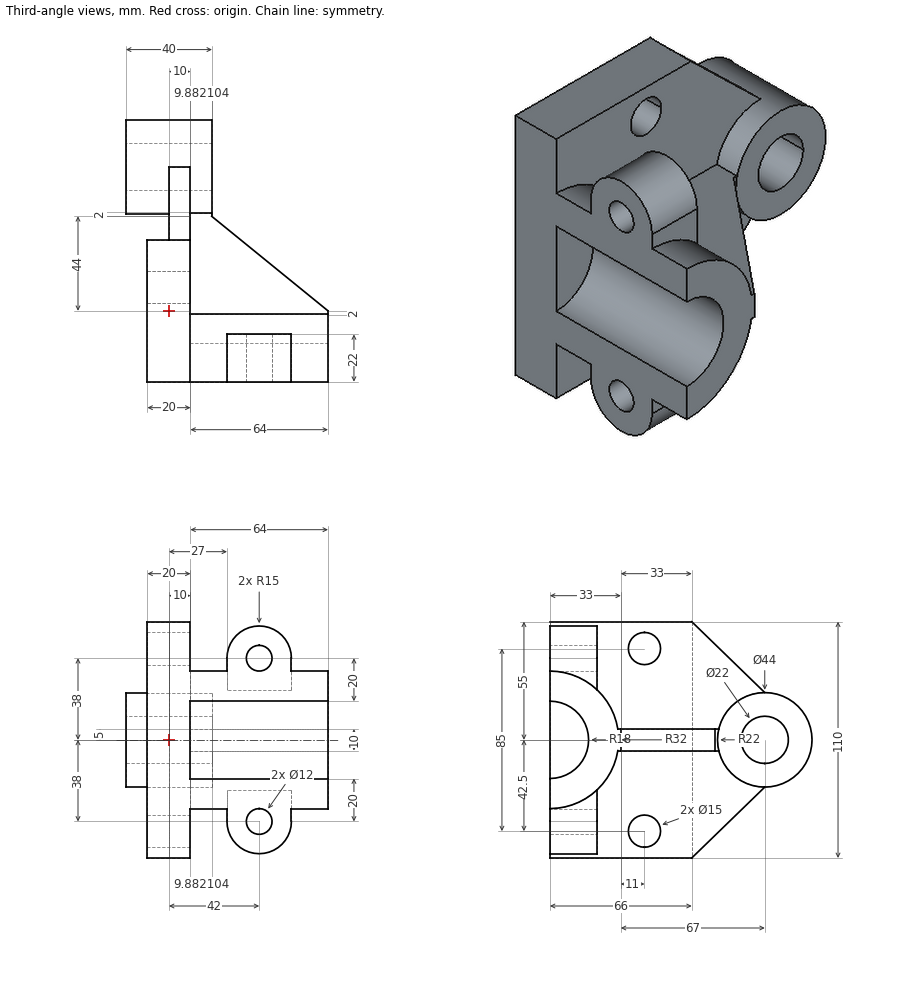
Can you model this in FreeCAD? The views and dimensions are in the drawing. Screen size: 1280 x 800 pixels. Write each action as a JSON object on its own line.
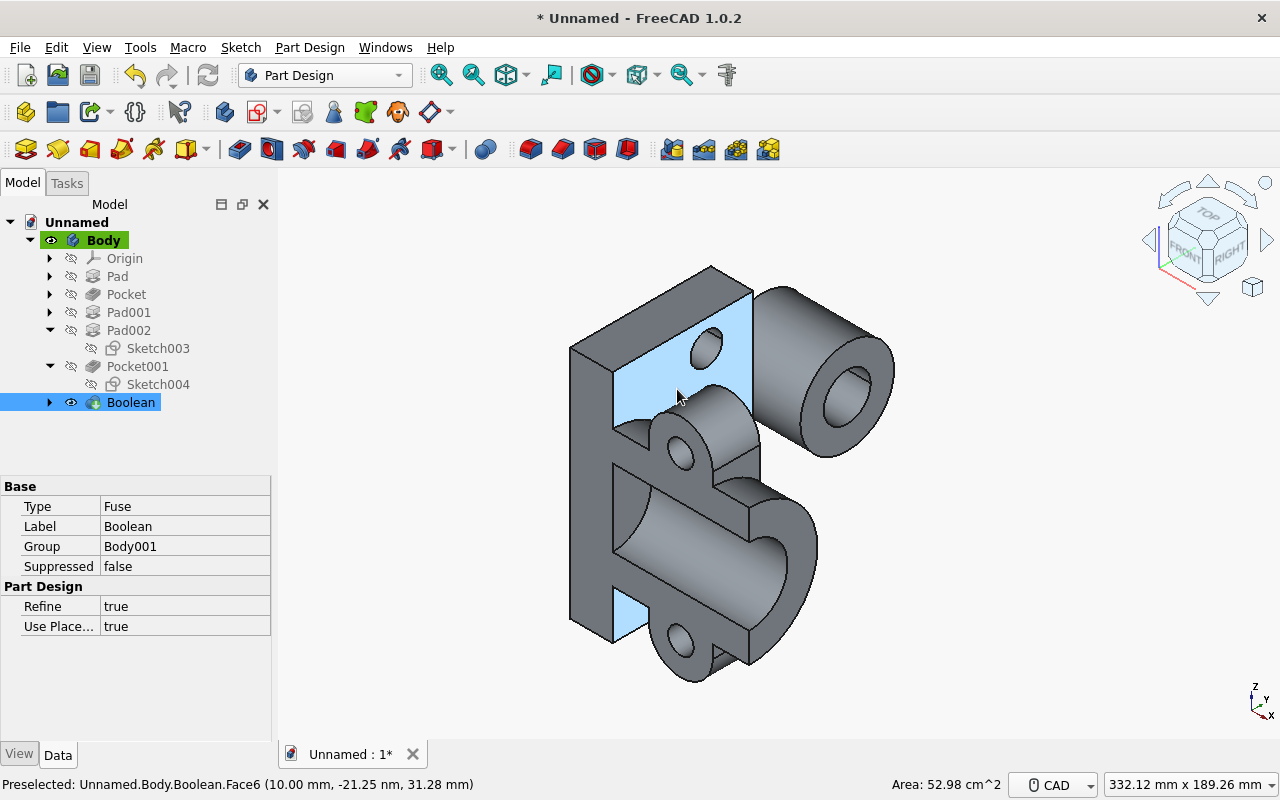
{"action": "left_click", "coordinate": [258, 112]}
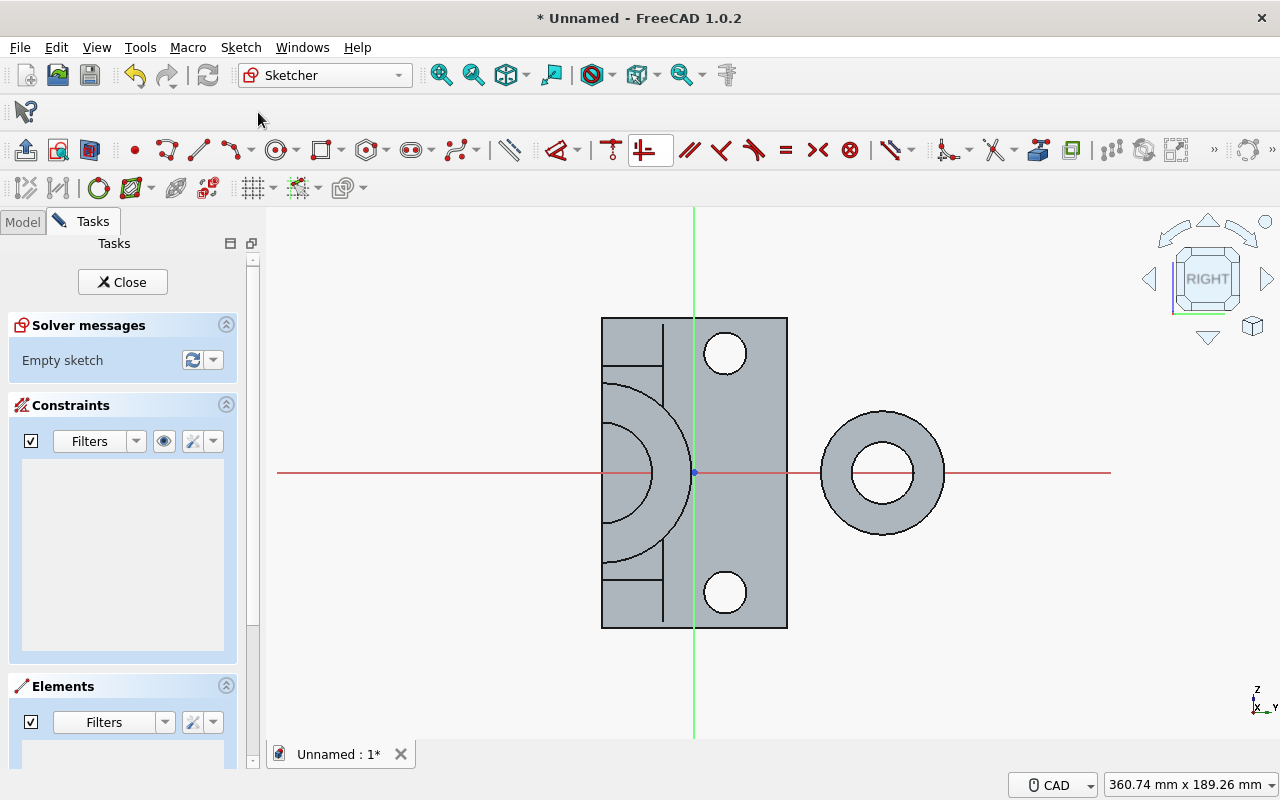
{"action": "left_click", "coordinate": [168, 150]}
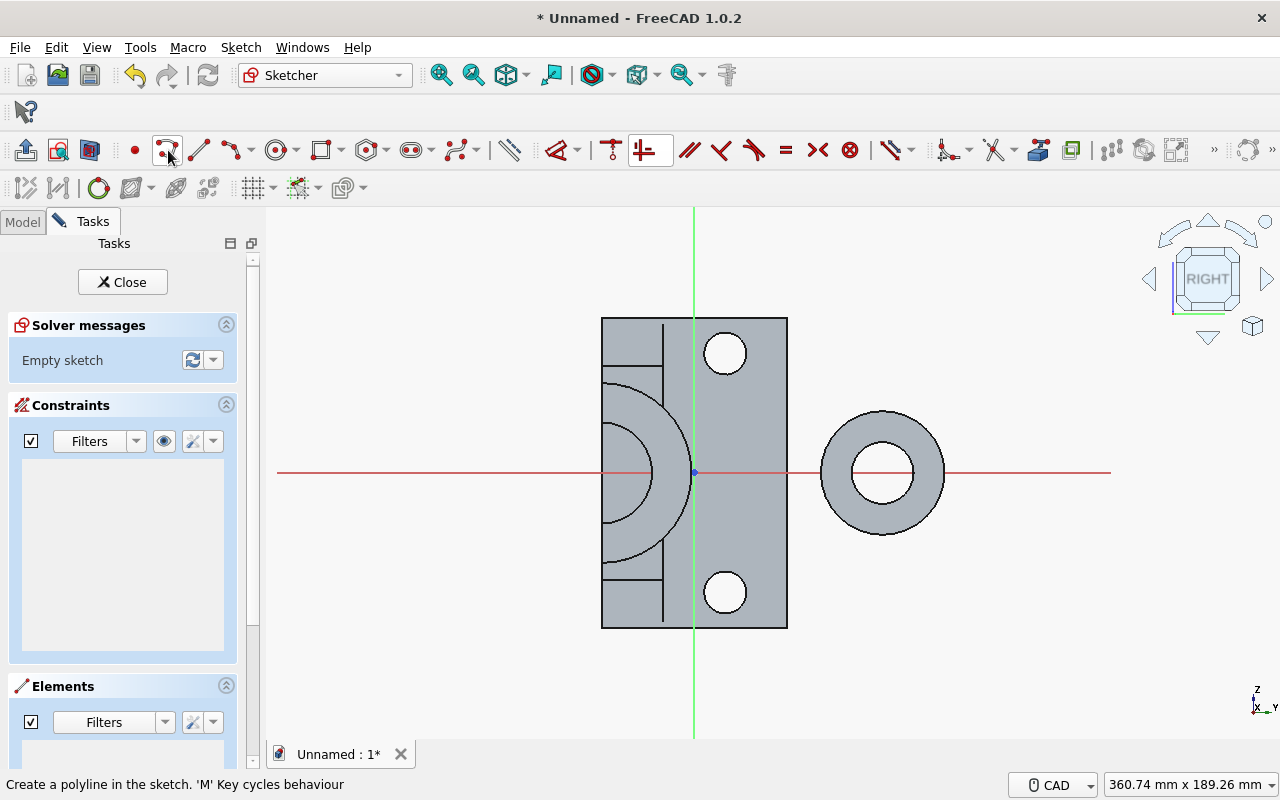
{"action": "left_click", "coordinate": [883, 411]}
{"action": "left_click", "coordinate": [787, 318]}
{"action": "left_click", "coordinate": [787, 628]}
{"action": "left_click", "coordinate": [883, 535]}
{"action": "right_click", "coordinate": [883, 535]}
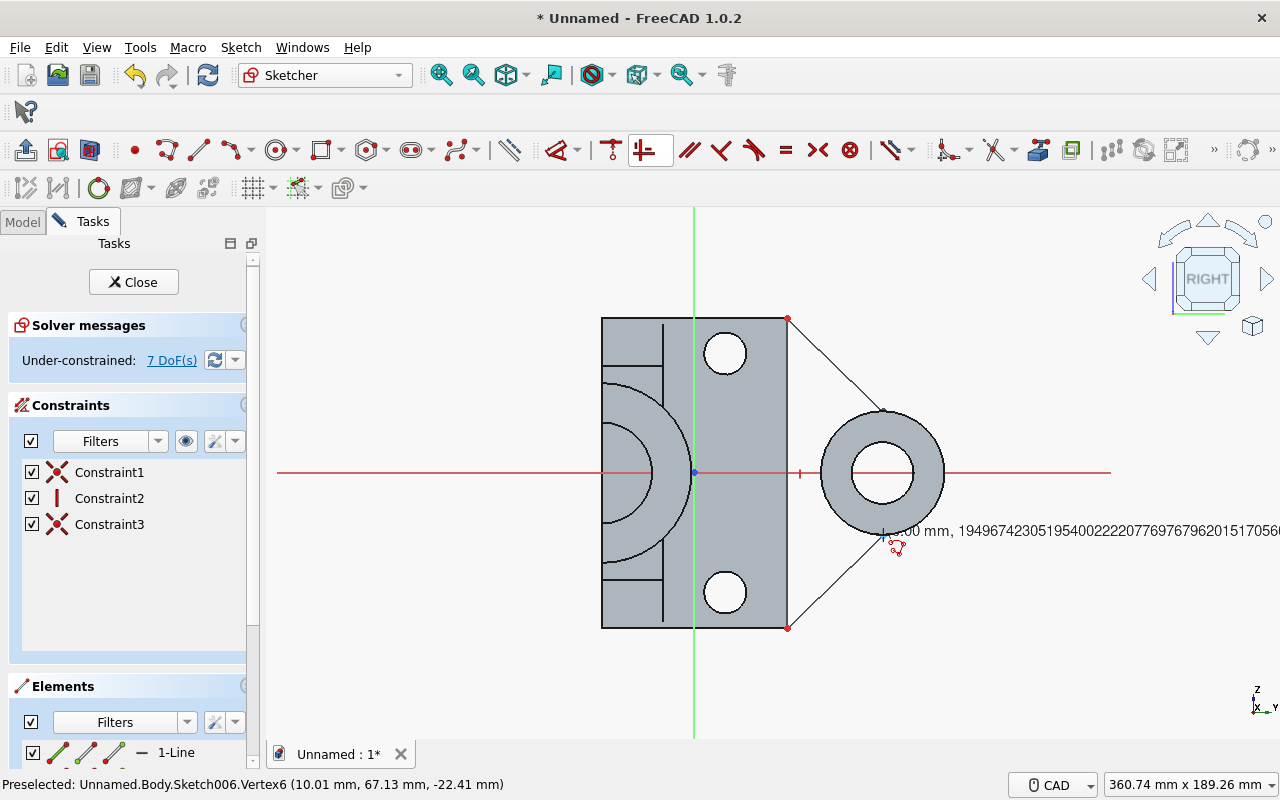
{"action": "left_click", "coordinate": [232, 150]}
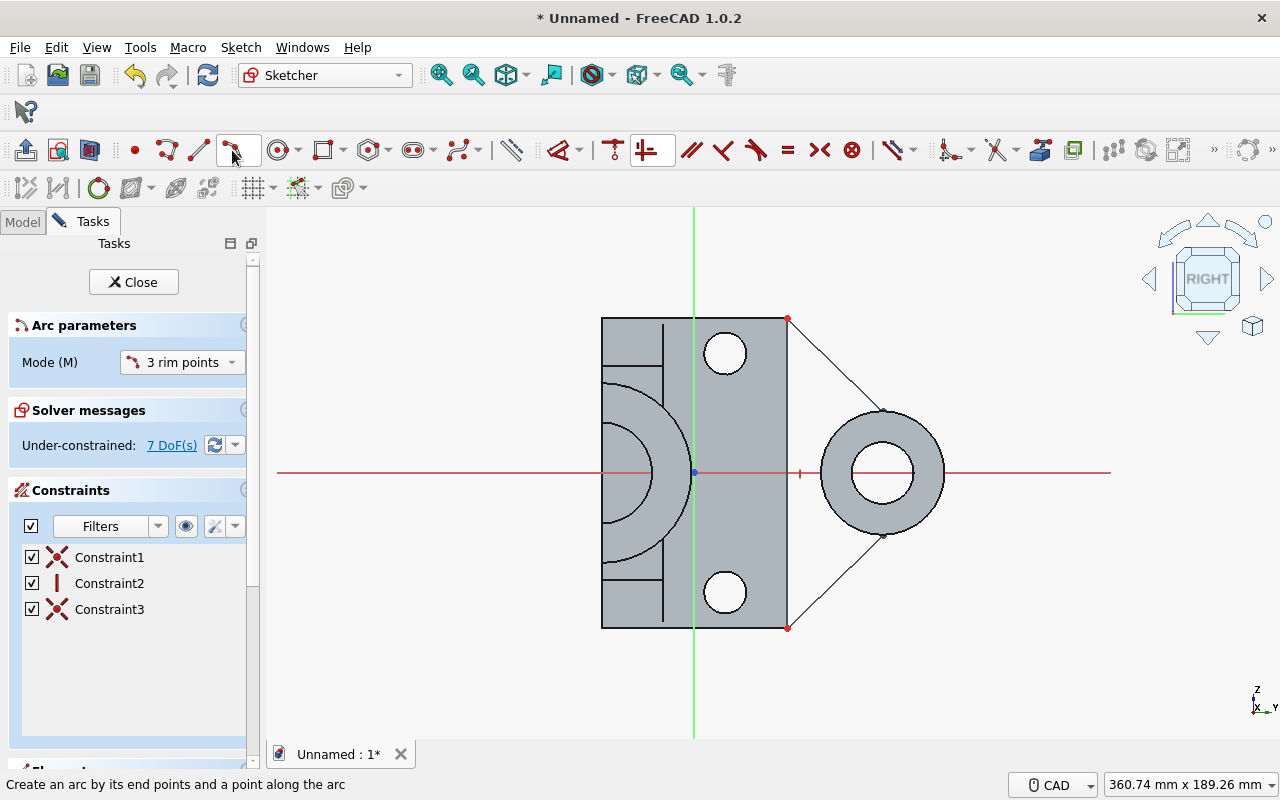
{"action": "left_click", "coordinate": [883, 536]}
{"action": "left_click", "coordinate": [883, 412]}
{"action": "left_click", "coordinate": [824, 454]}
{"action": "key", "text": "Escape"}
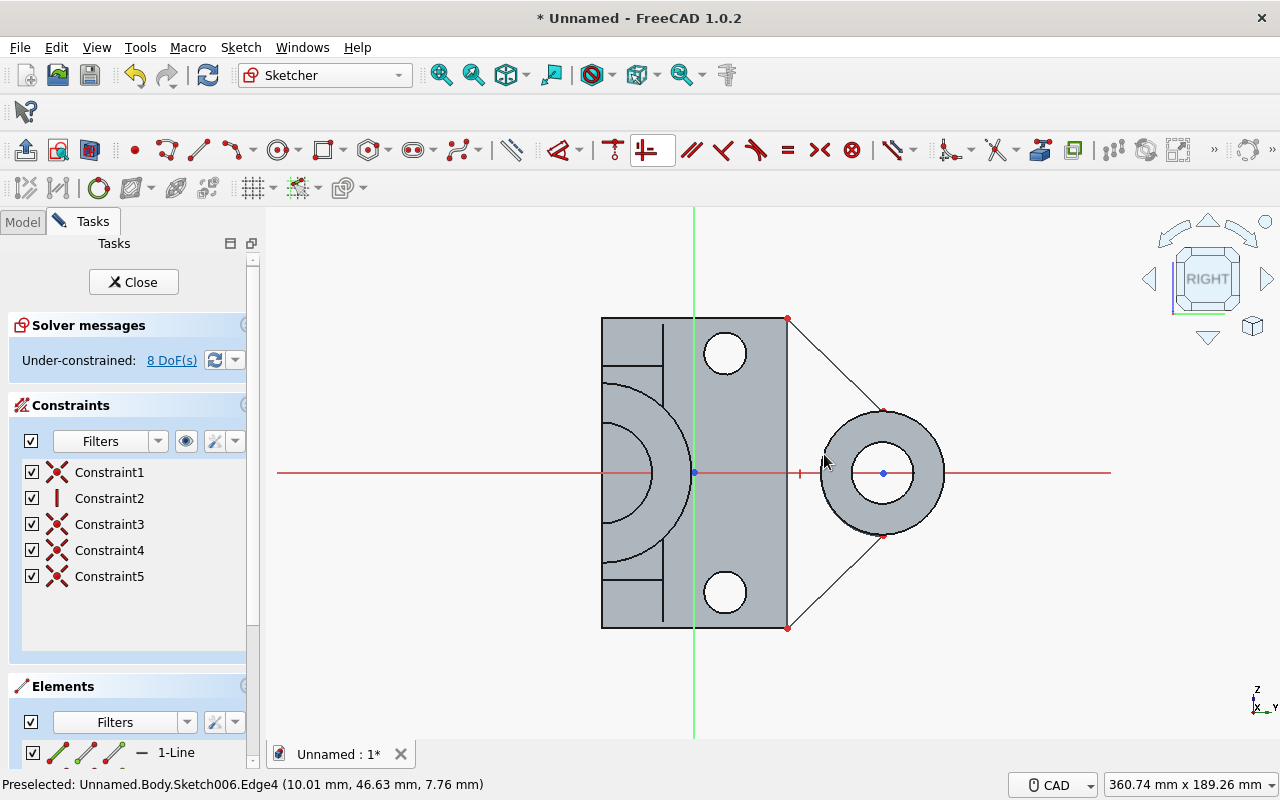
{"action": "left_click", "coordinate": [883, 474]}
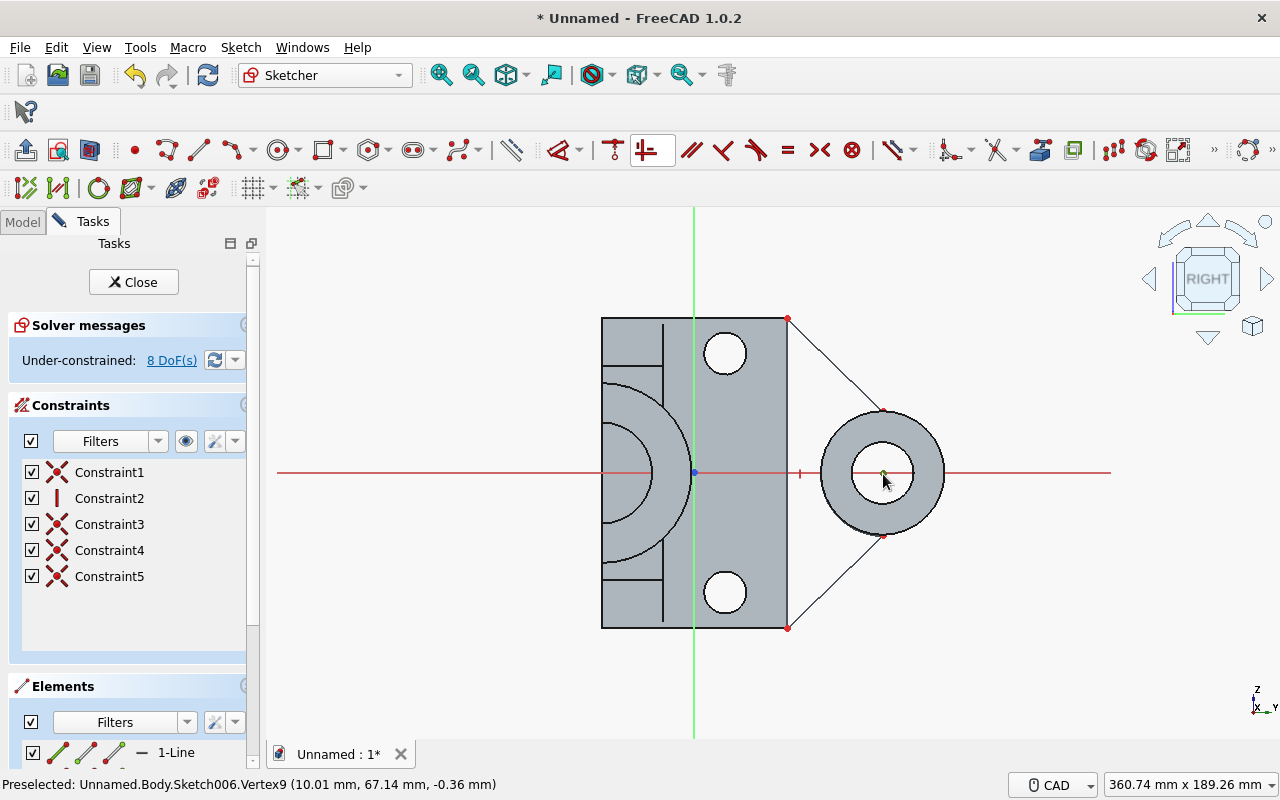
{"action": "left_click", "coordinate": [353, 473]}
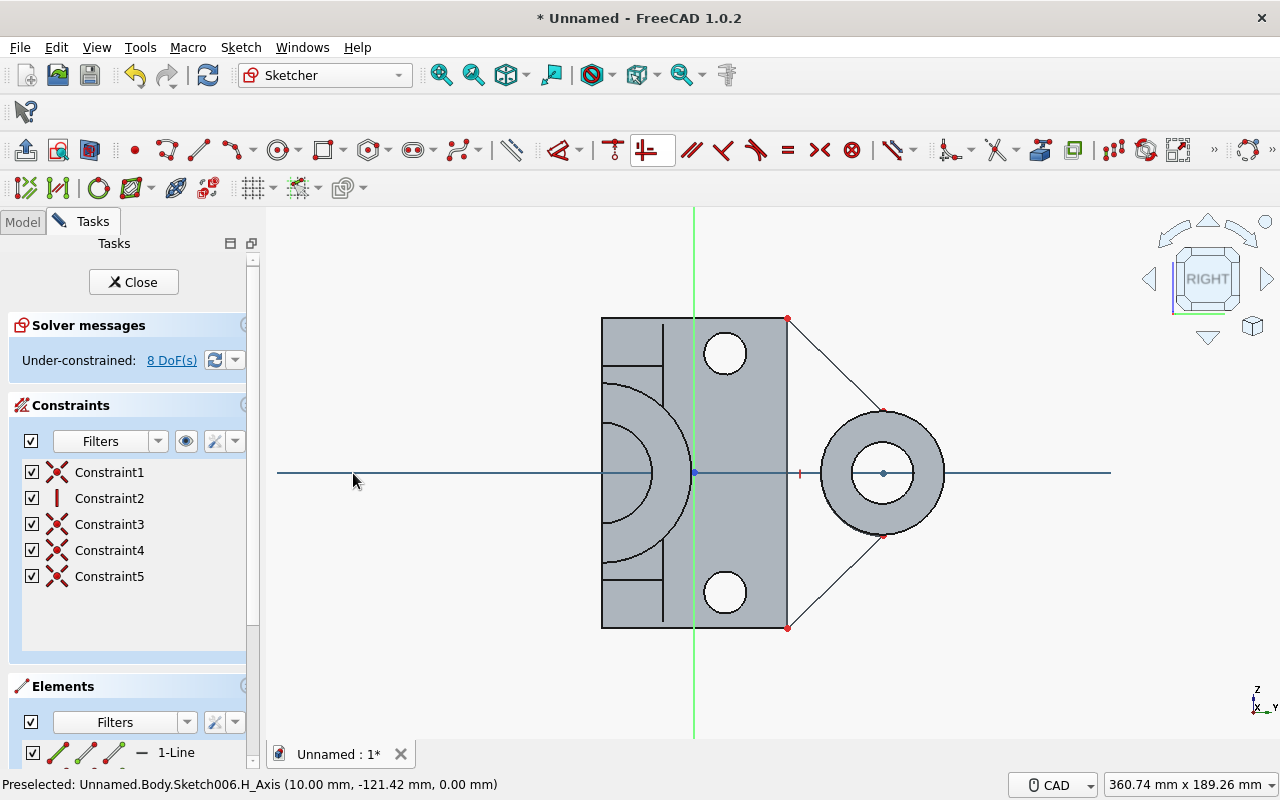
{"action": "left_click", "coordinate": [614, 150]}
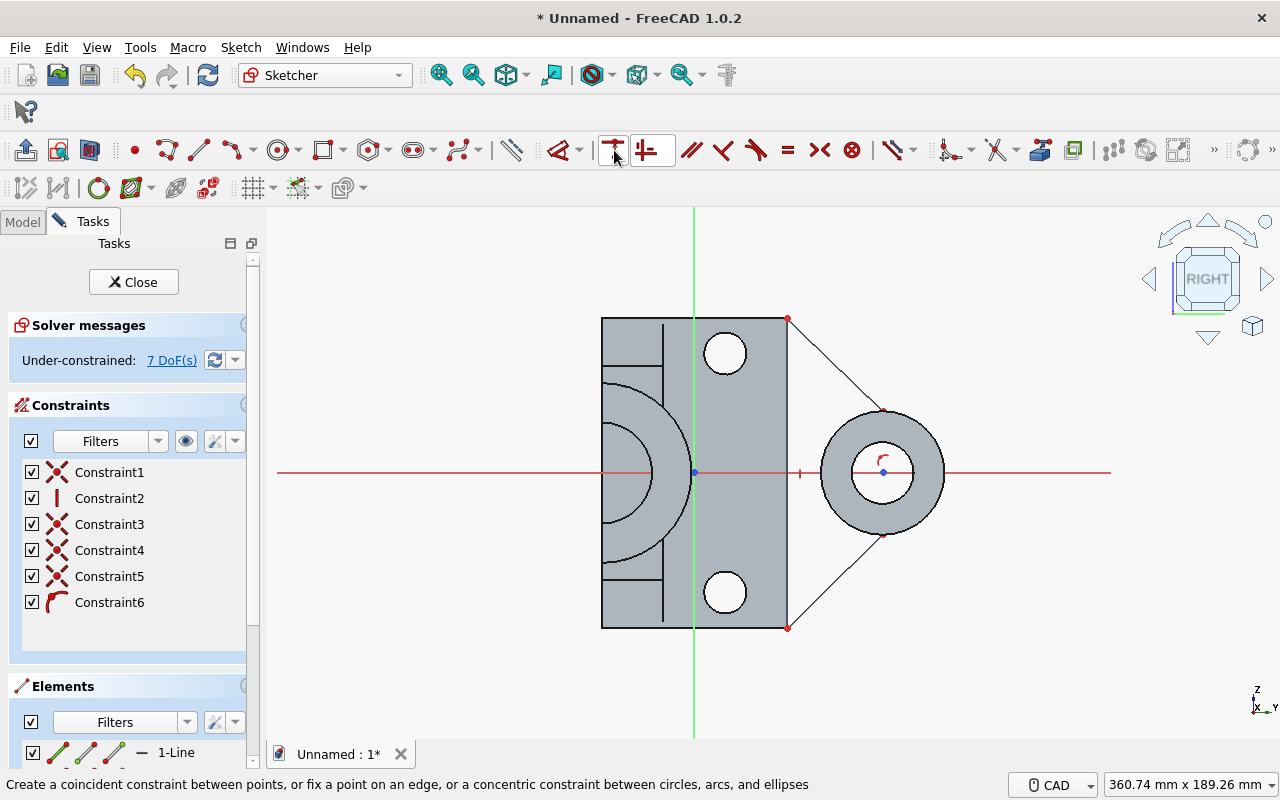
{"action": "left_click", "coordinate": [558, 150]}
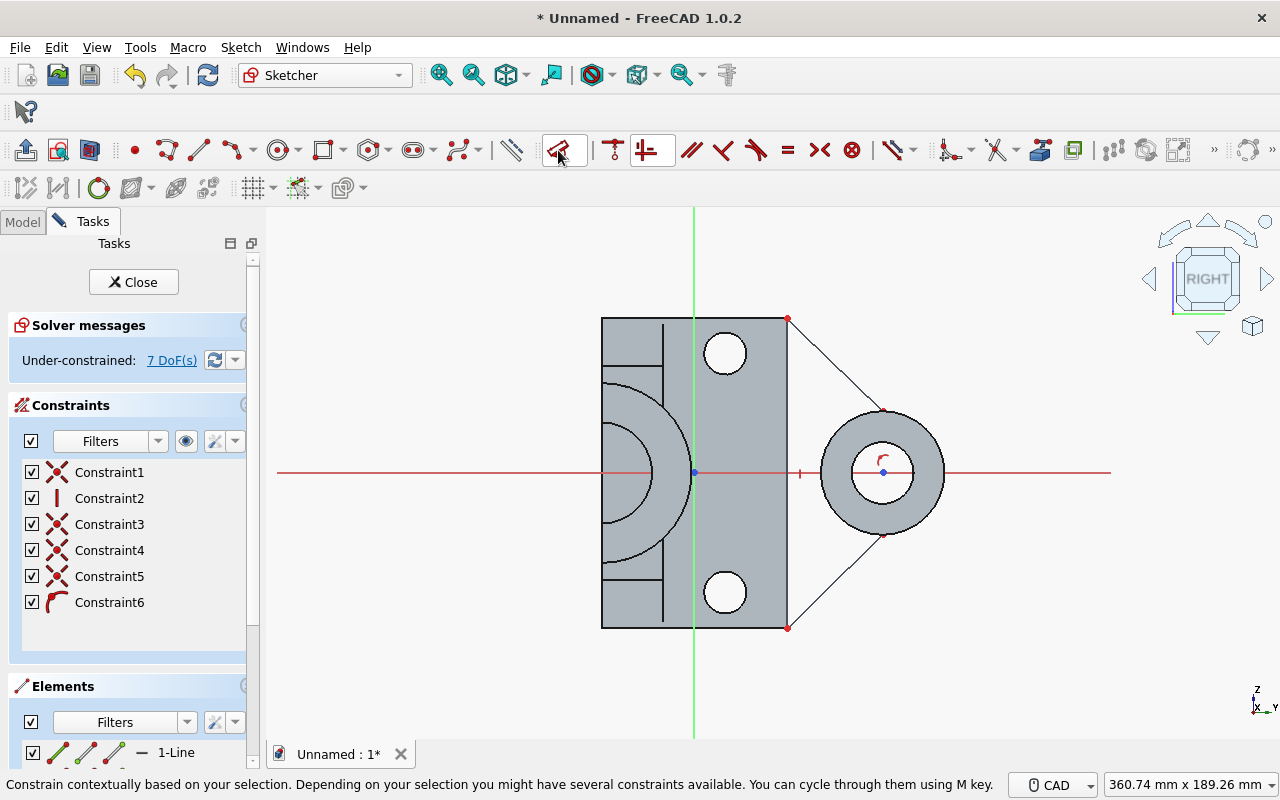
{"action": "left_click", "coordinate": [833, 437]}
{"action": "left_click", "coordinate": [807, 418]}